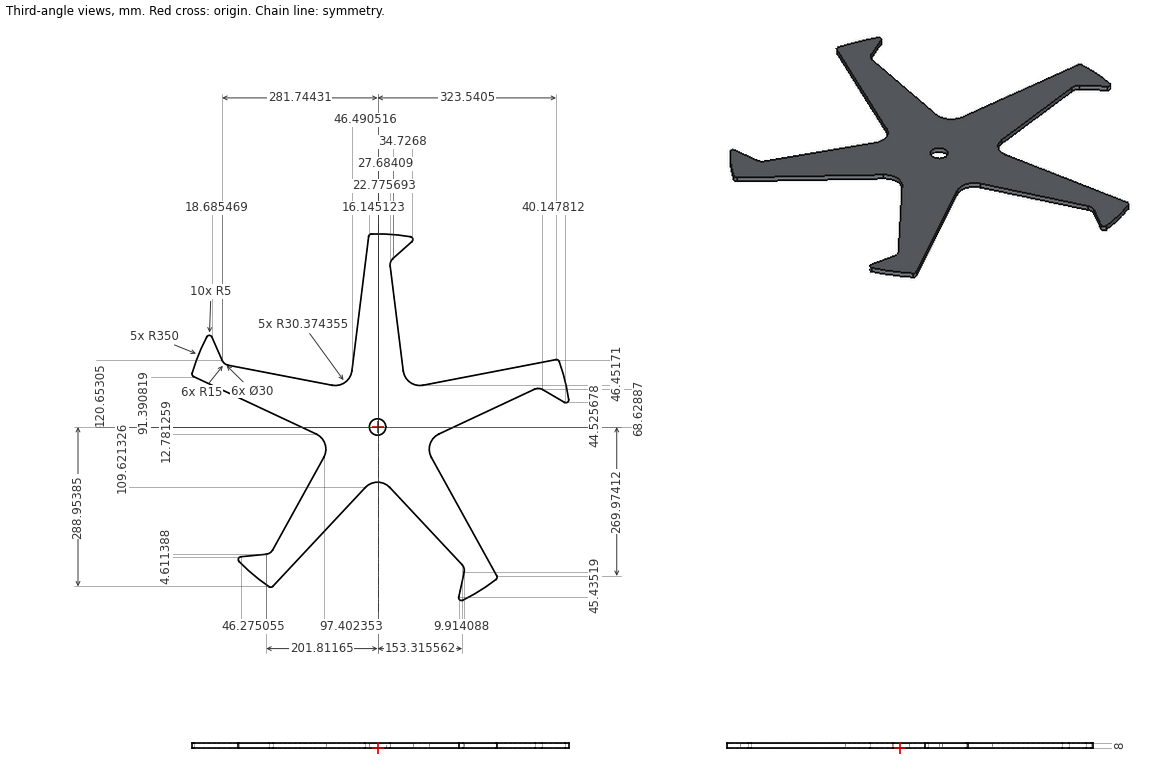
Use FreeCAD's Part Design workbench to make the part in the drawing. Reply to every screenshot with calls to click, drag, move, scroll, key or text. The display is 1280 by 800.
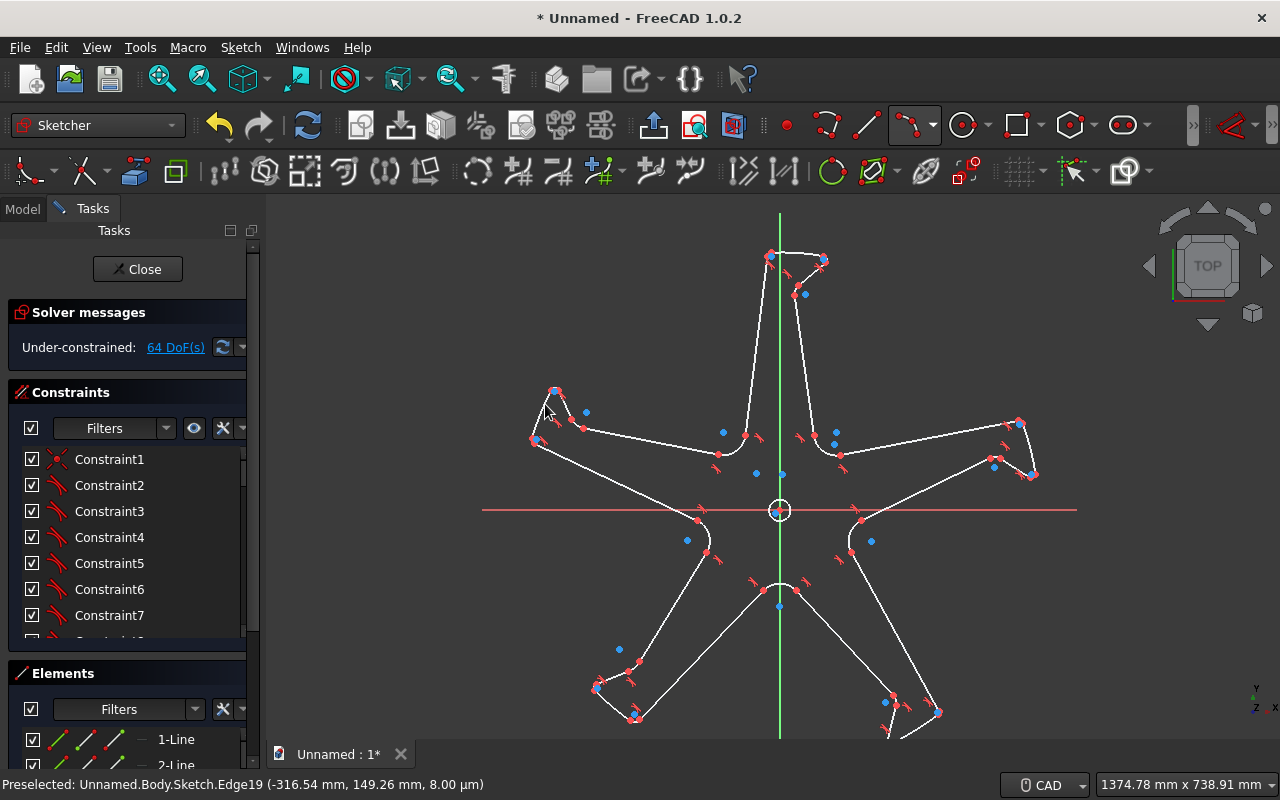
scroll(780, 500, up, 2)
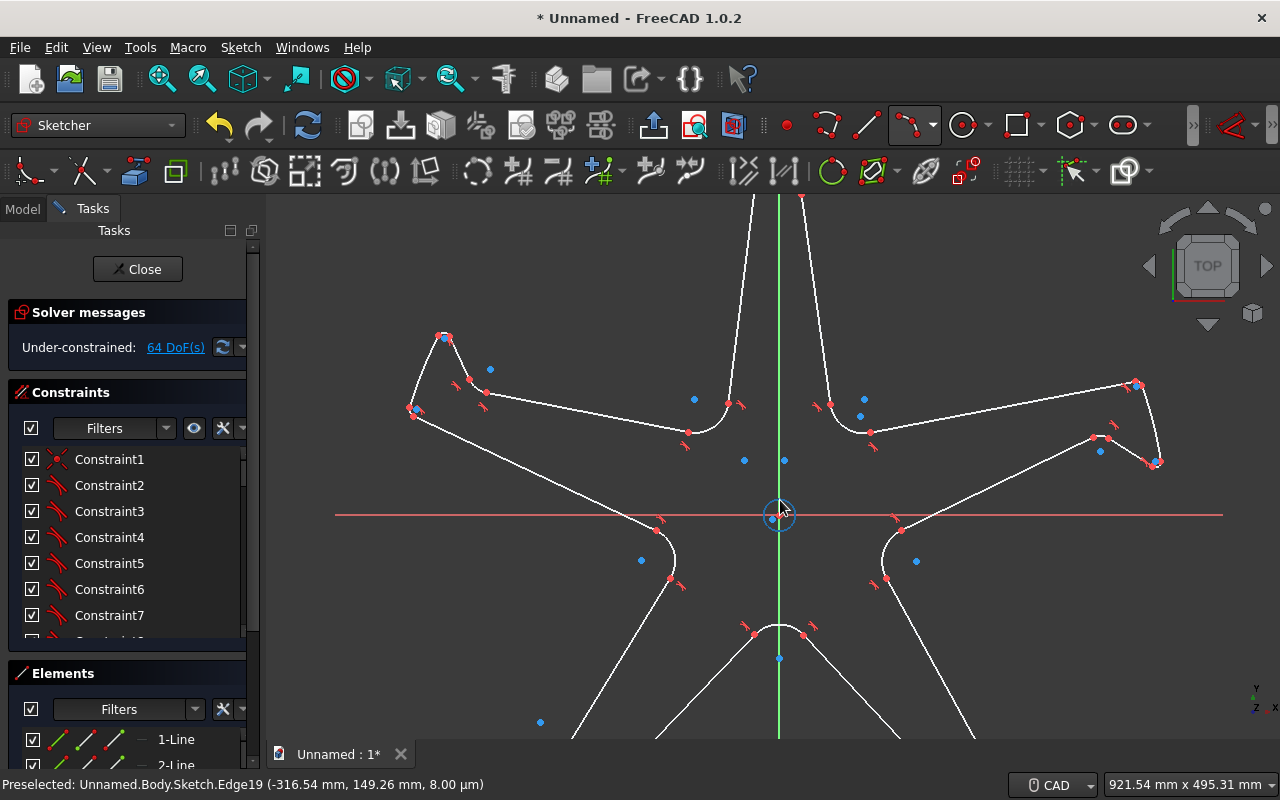
click(780, 499)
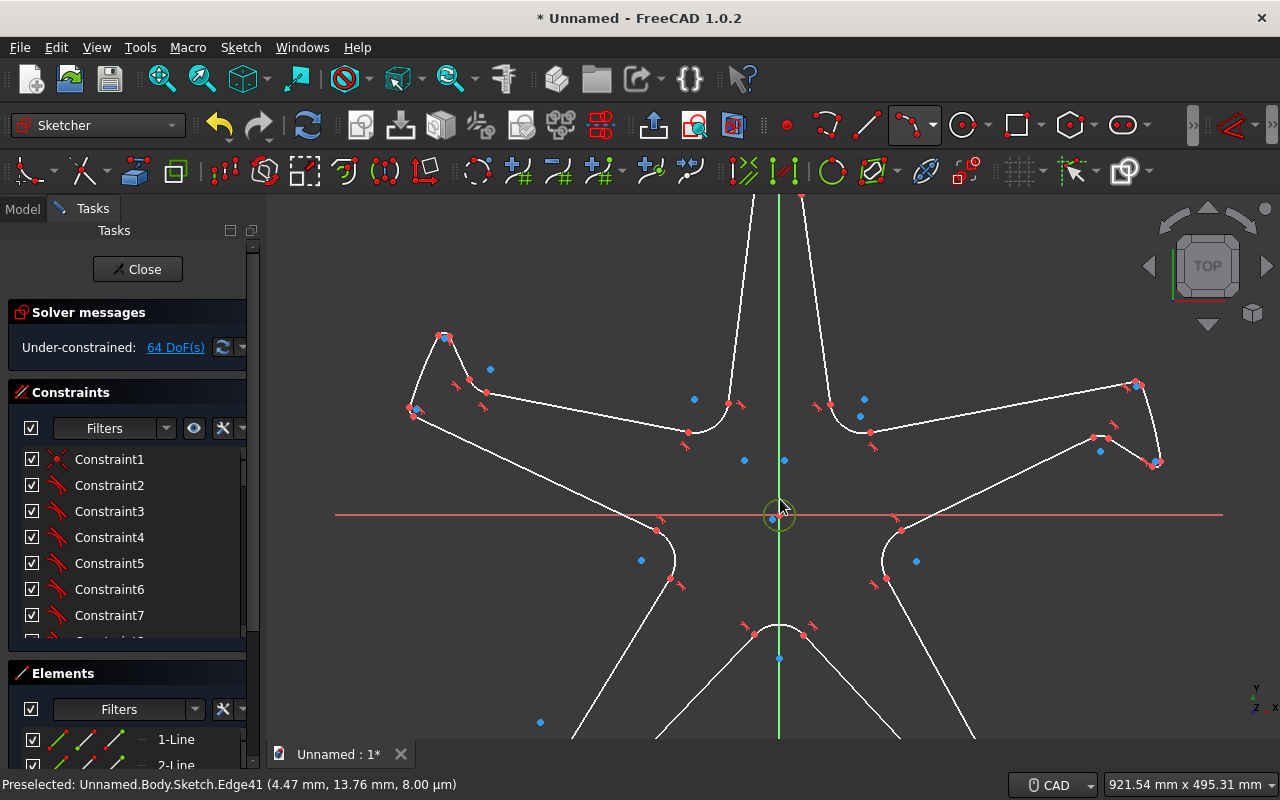
scroll(639, 443, down, 4)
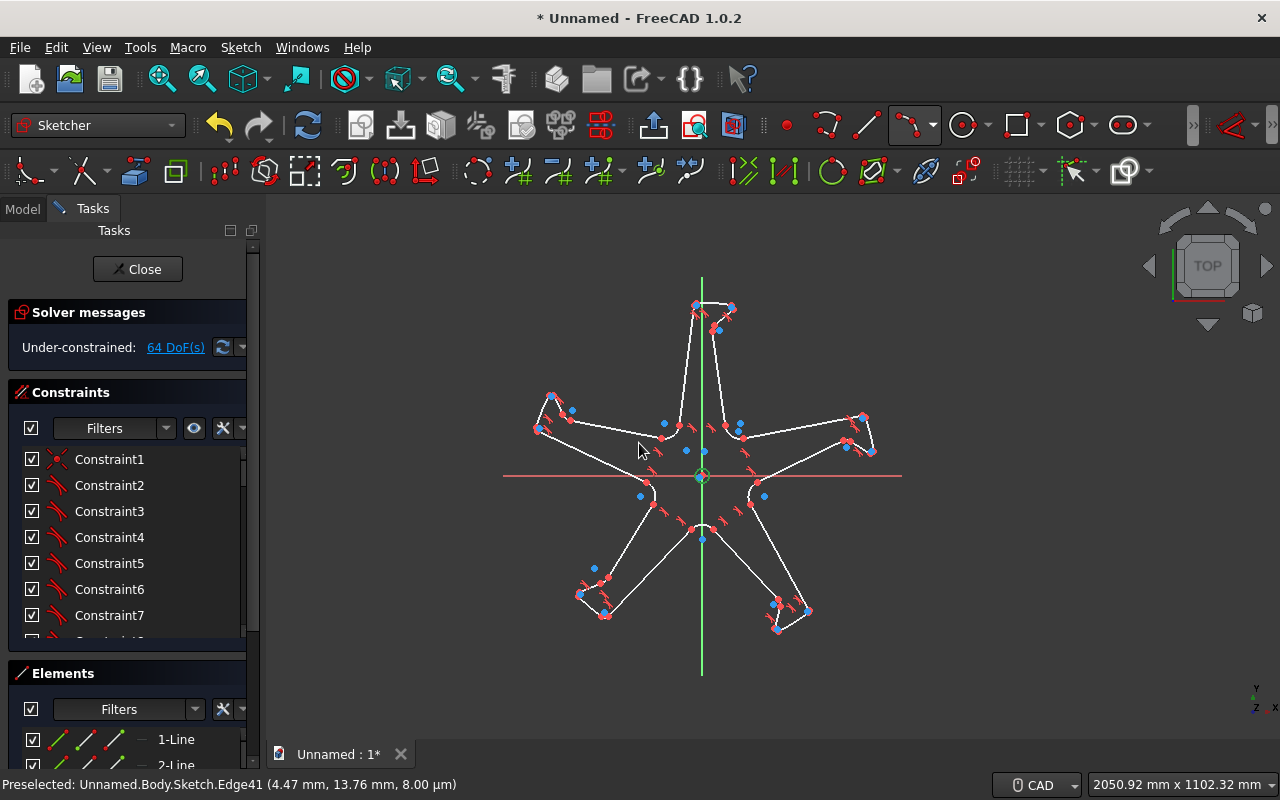
scroll(585, 603, up, 2)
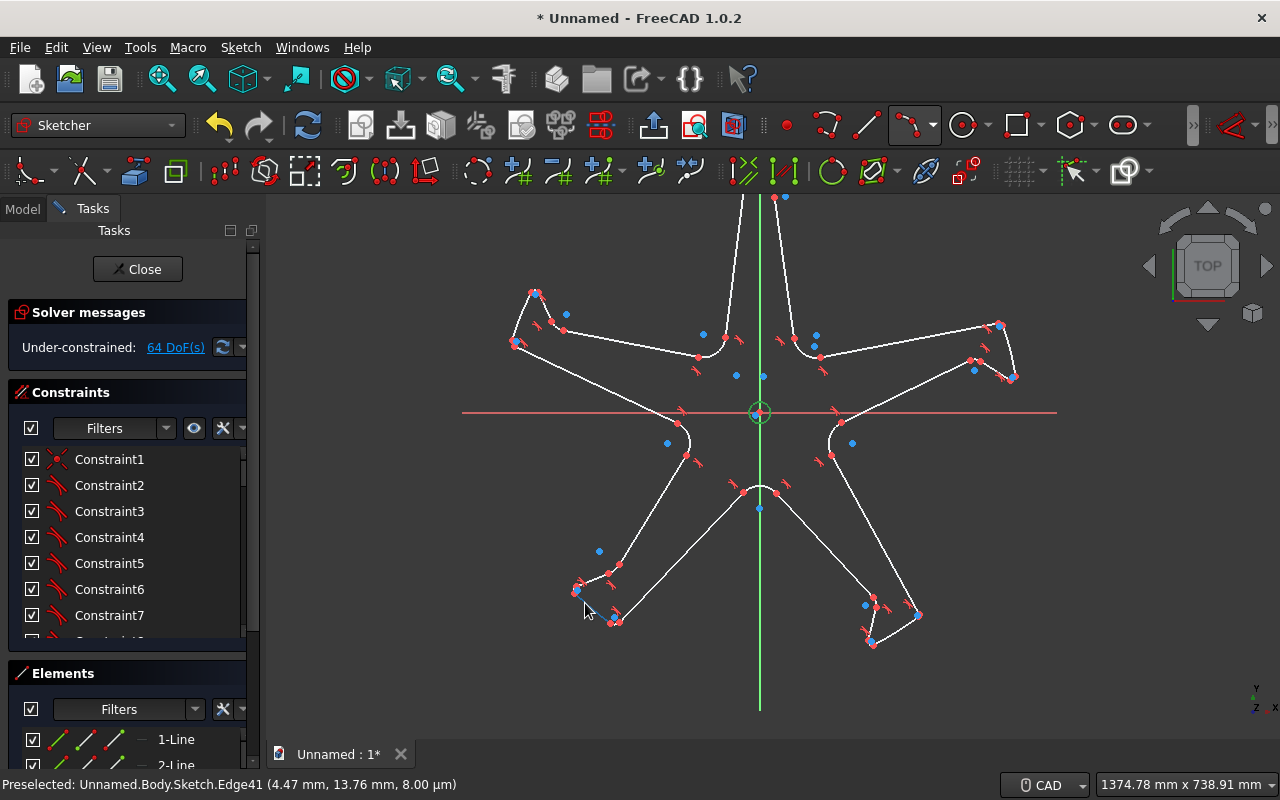
click(585, 603)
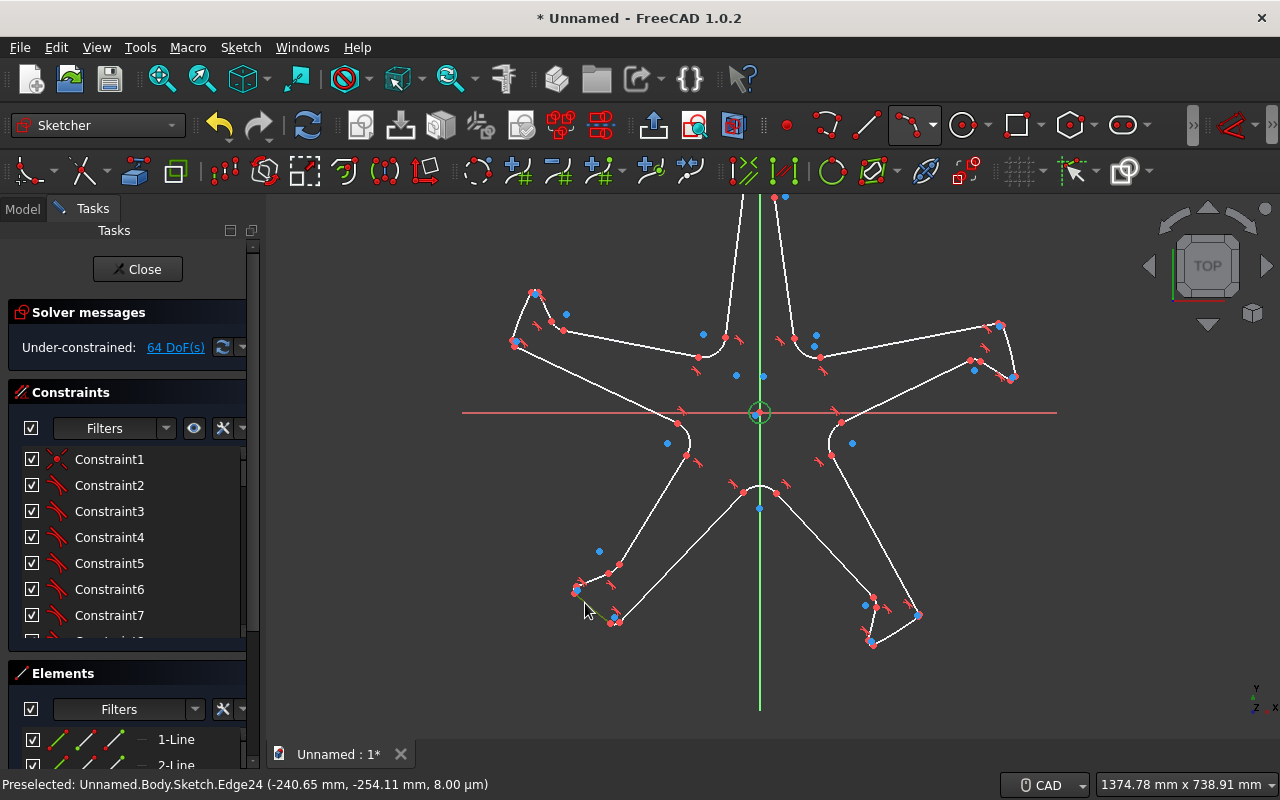
key(c)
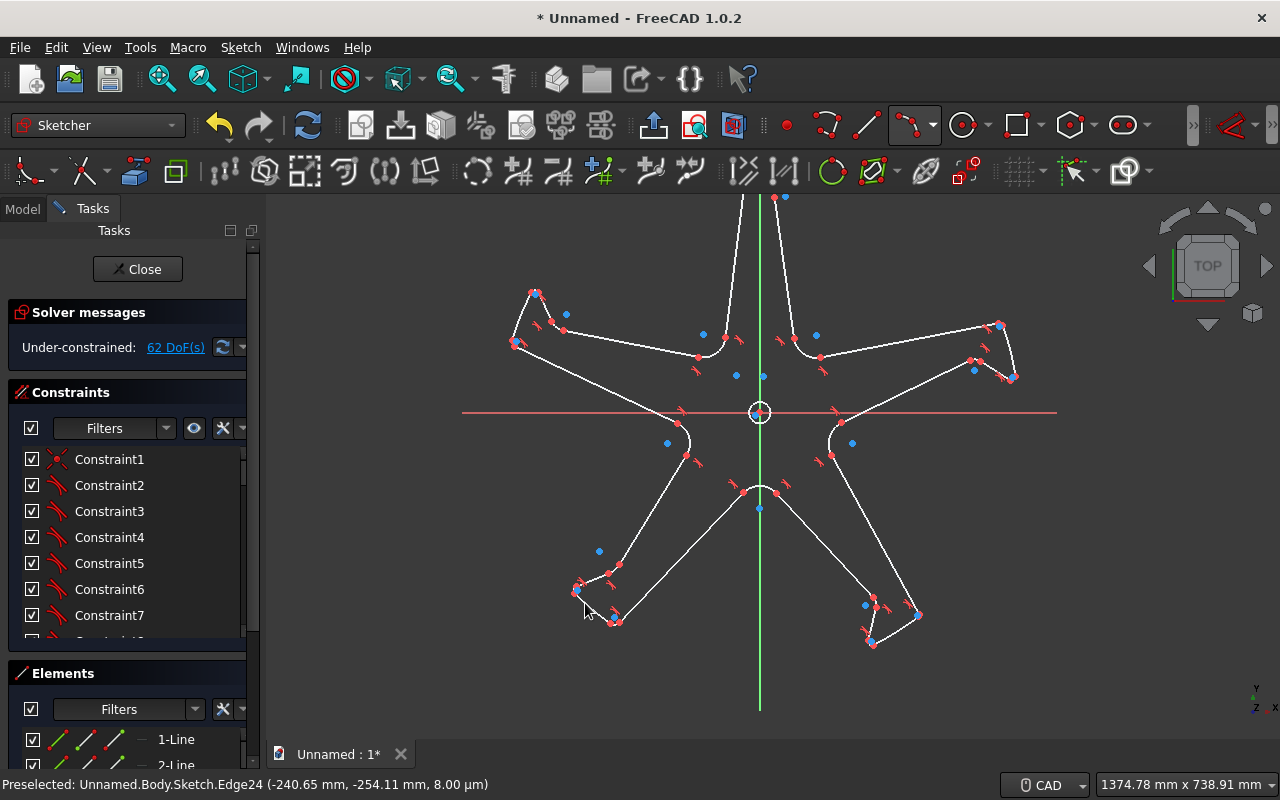
scroll(760, 402, up, 2)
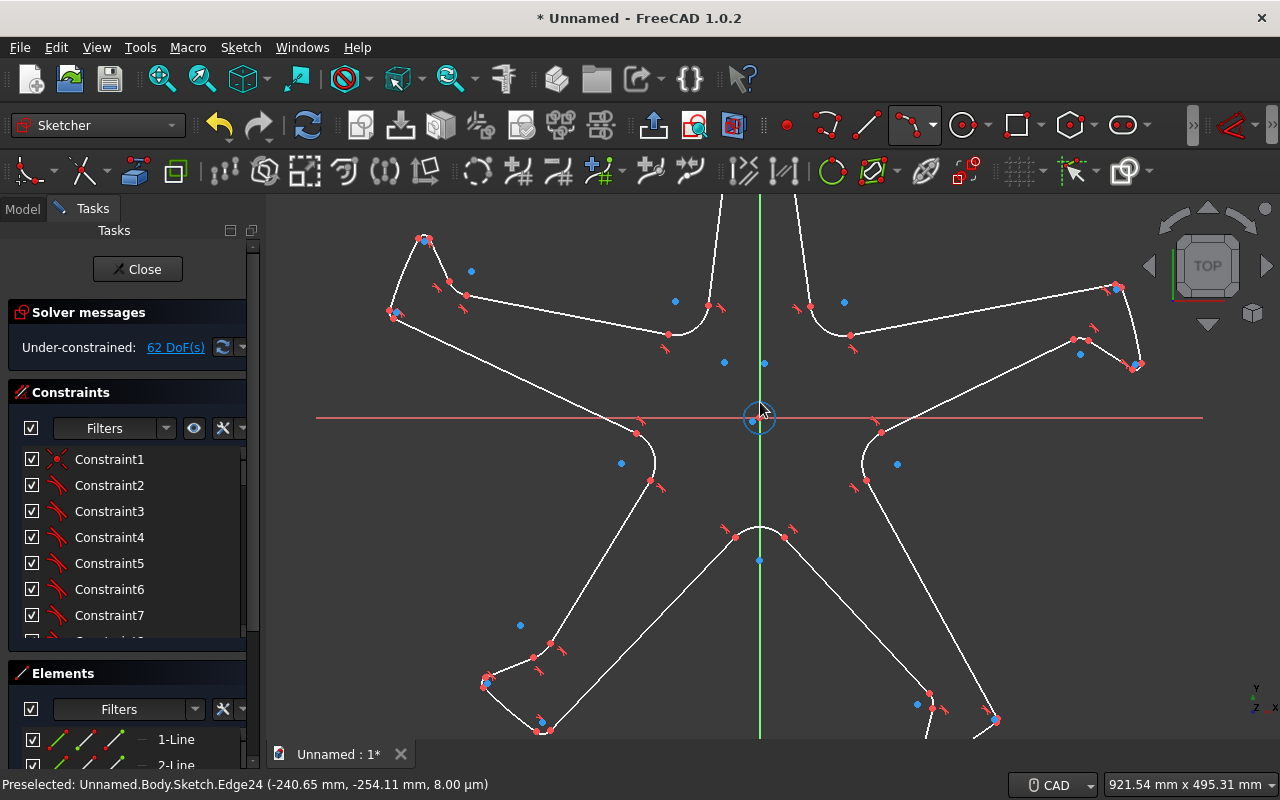
click(760, 402)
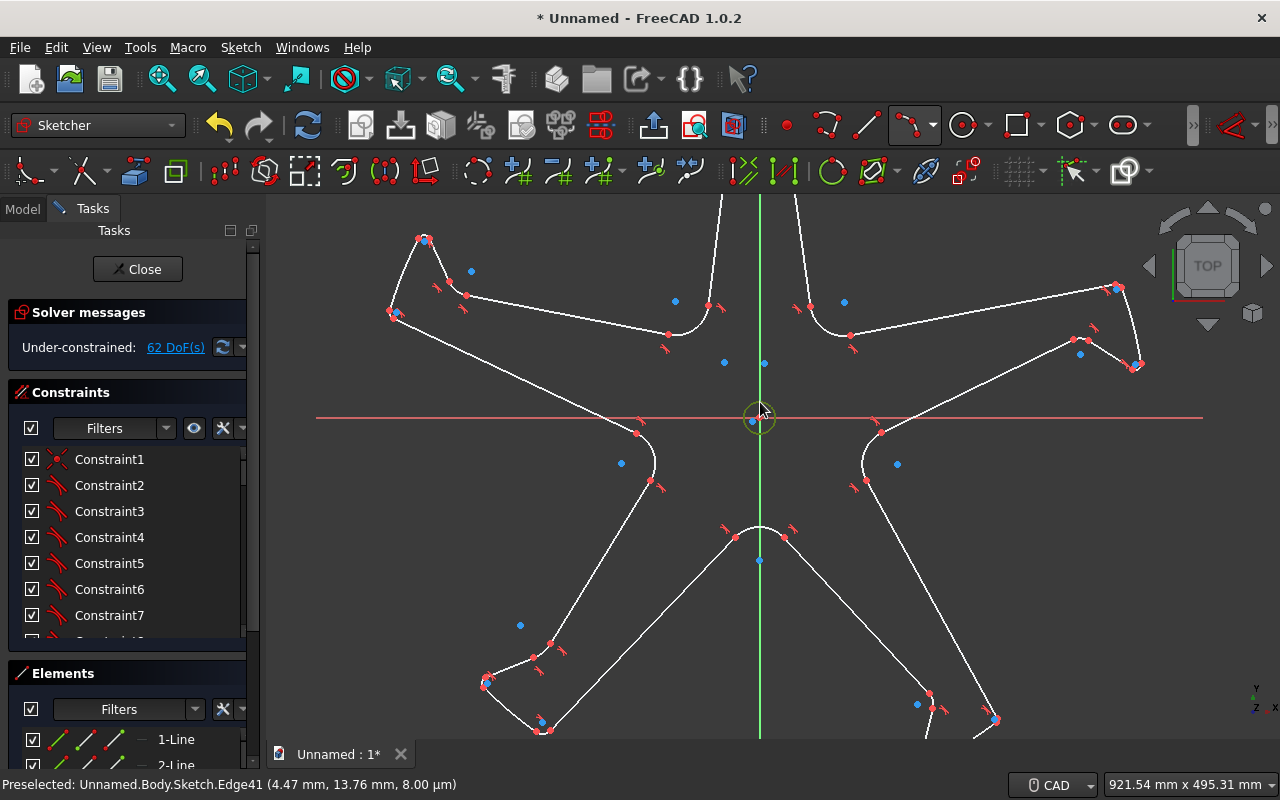
scroll(655, 522, down, 4)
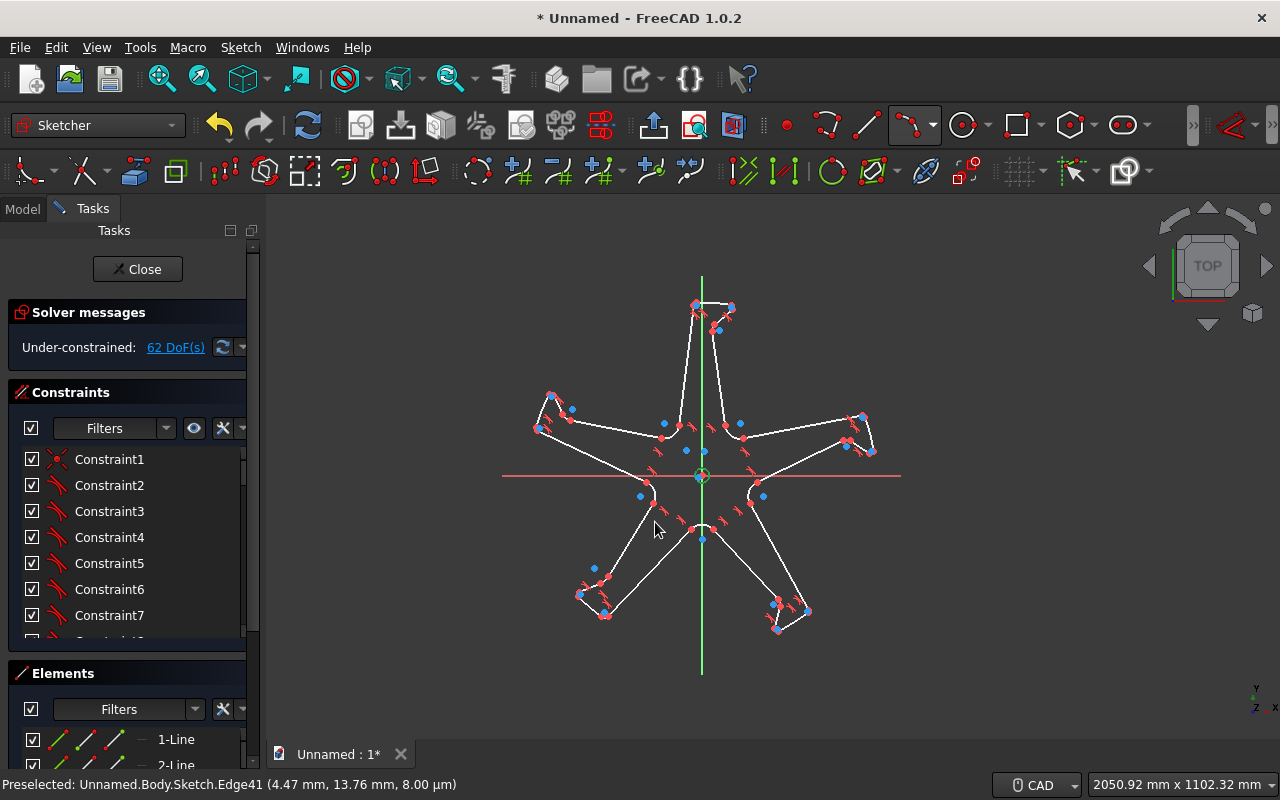
scroll(788, 626, up, 2)